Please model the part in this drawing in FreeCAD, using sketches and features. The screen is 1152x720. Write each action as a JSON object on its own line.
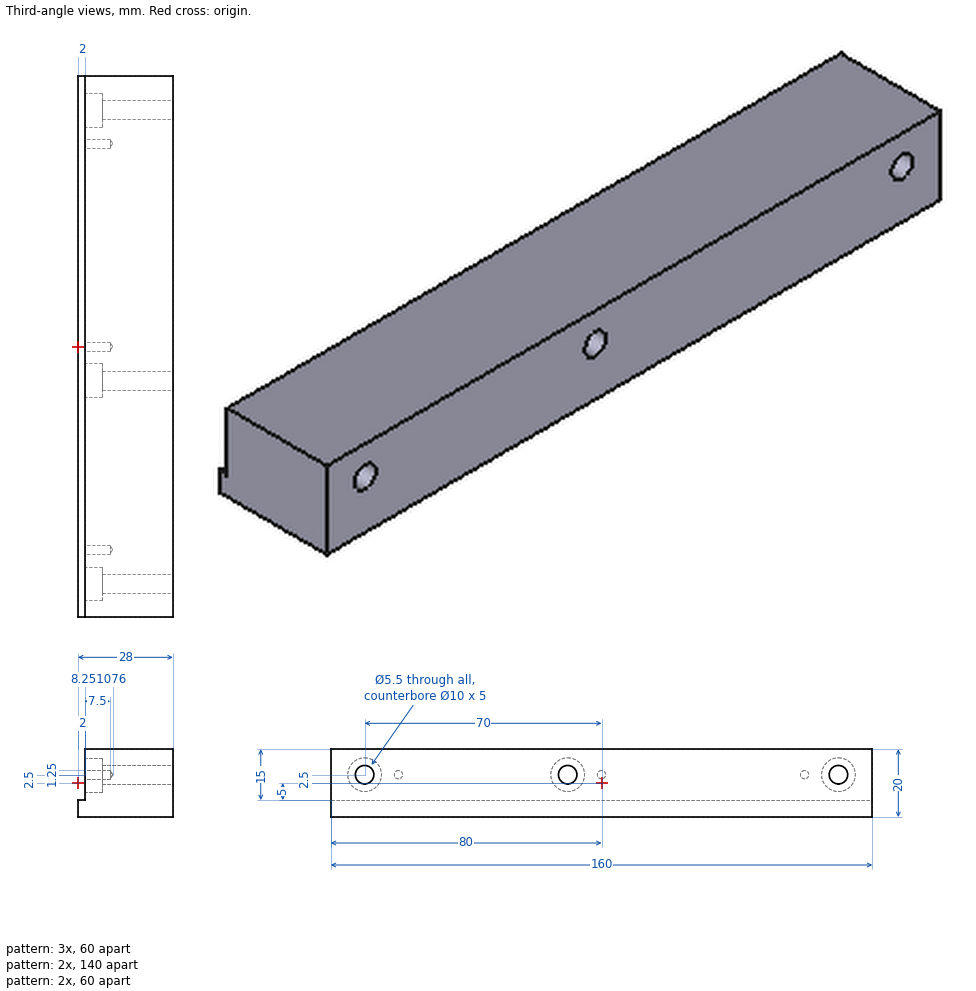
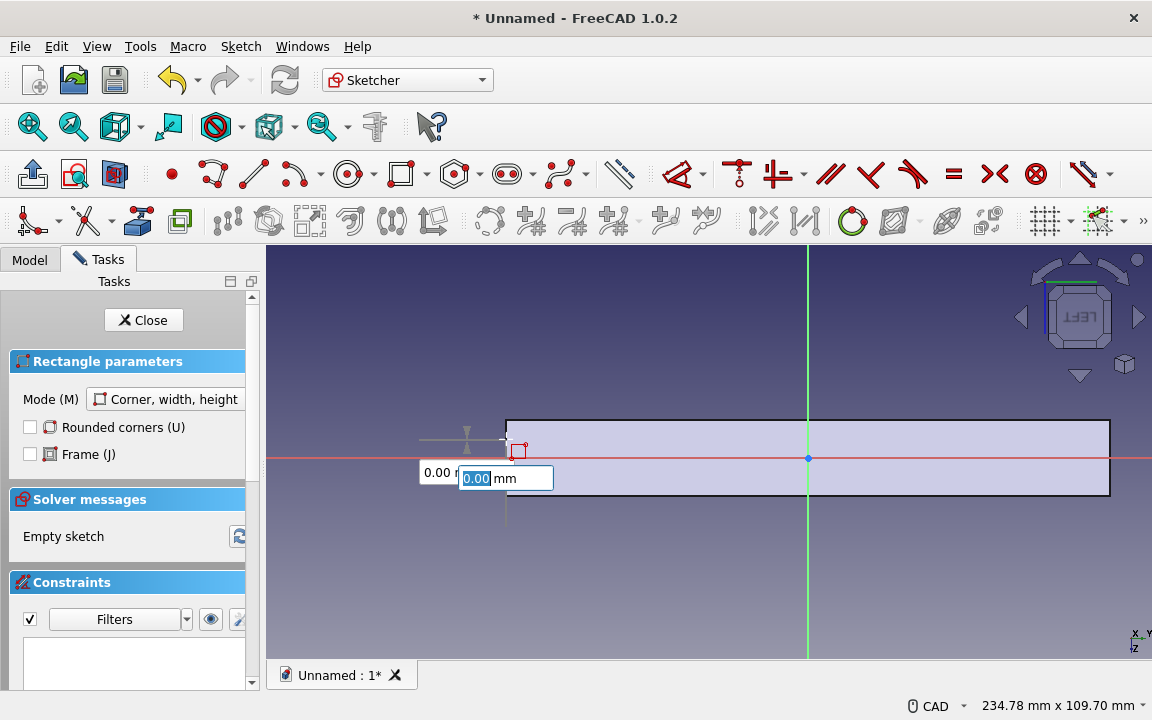
{"action": "scroll", "coordinate": [299, 420], "scroll_direction": "down", "scroll_amount": 2}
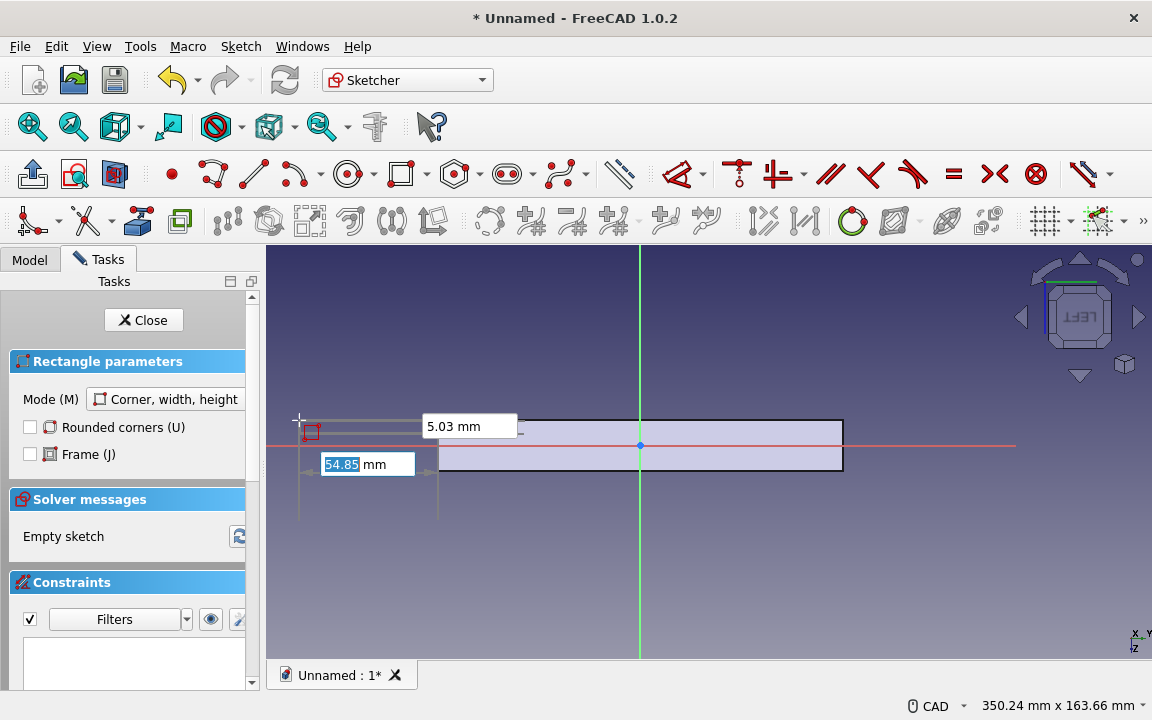
{"action": "left_click", "coordinate": [843, 471]}
{"action": "key", "text": "Escape"}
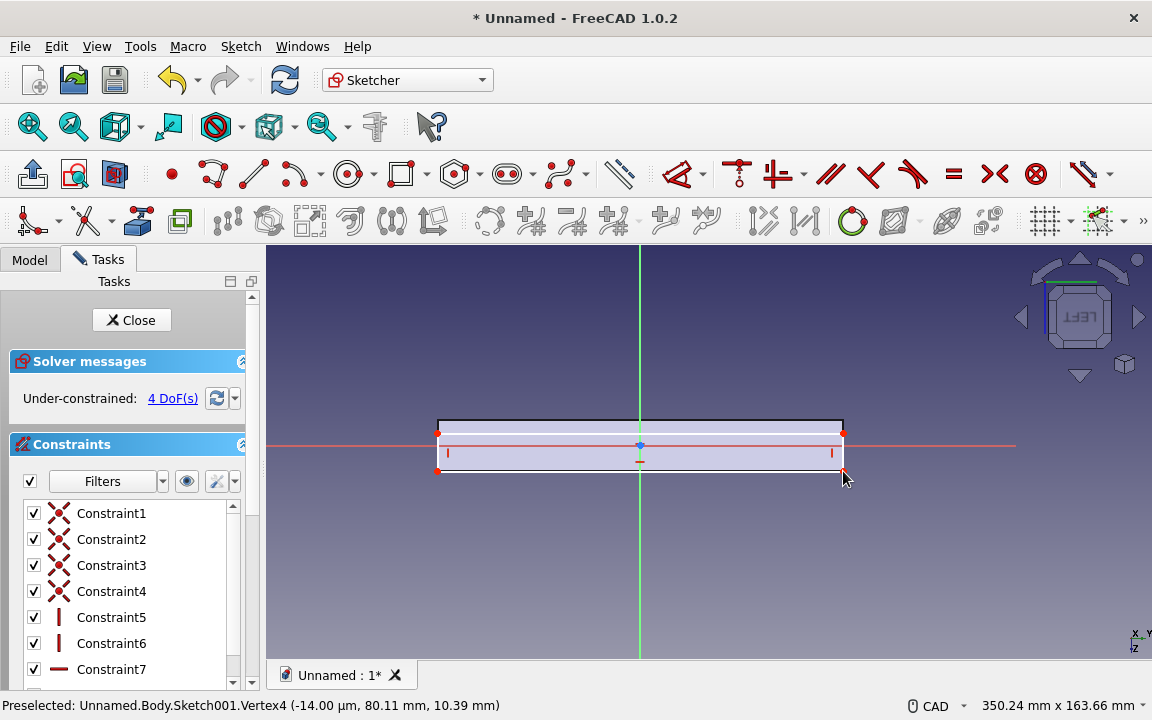
{"action": "key", "text": "d"}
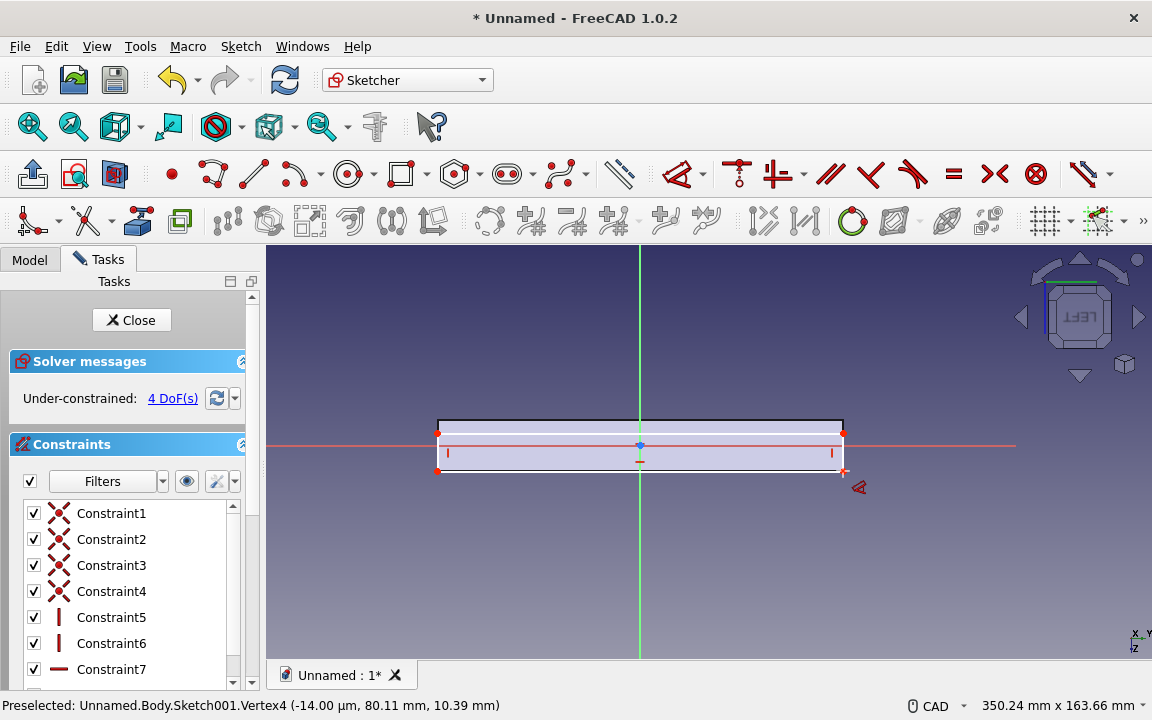
{"action": "left_click", "coordinate": [438, 445]}
{"action": "left_click", "coordinate": [404, 462]}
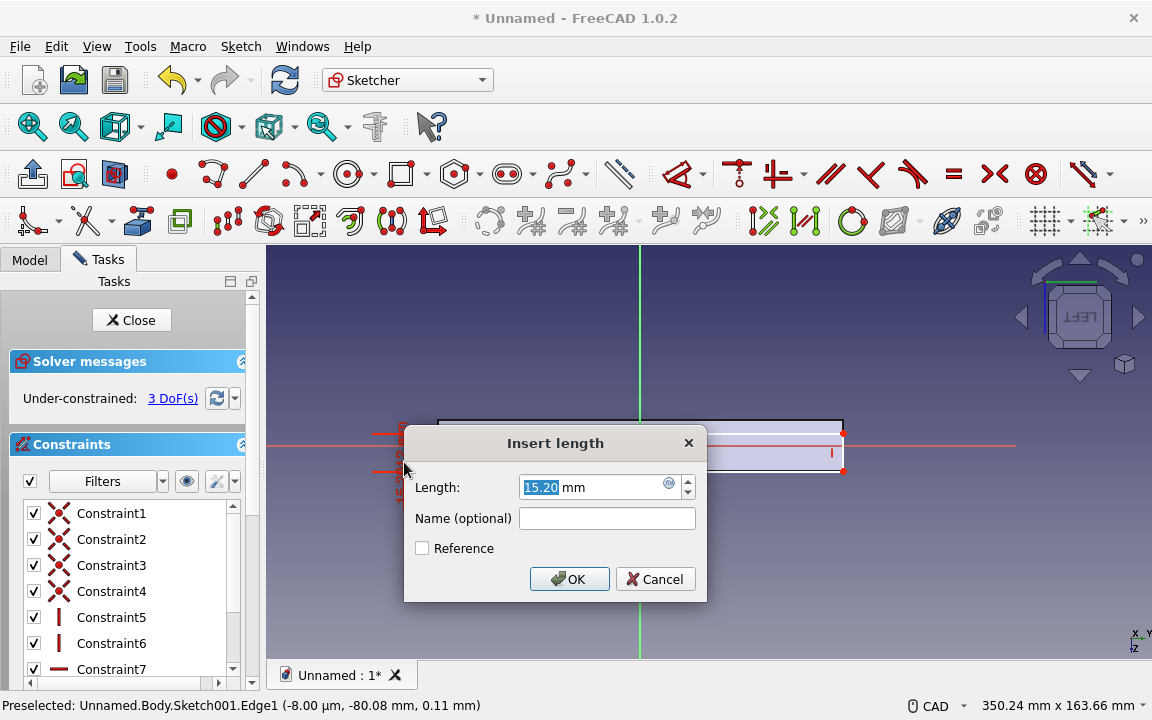
{"action": "type", "text": "15"}
{"action": "key", "text": "Return"}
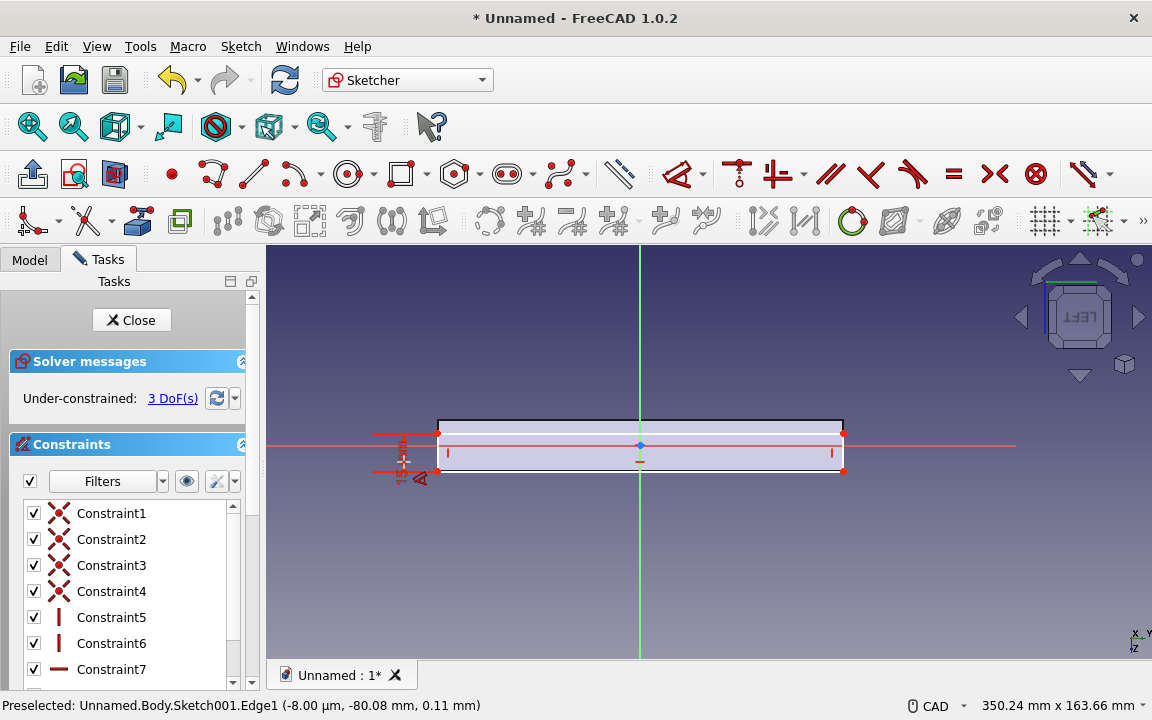
{"action": "scroll", "coordinate": [438, 434], "scroll_direction": "up", "scroll_amount": 6}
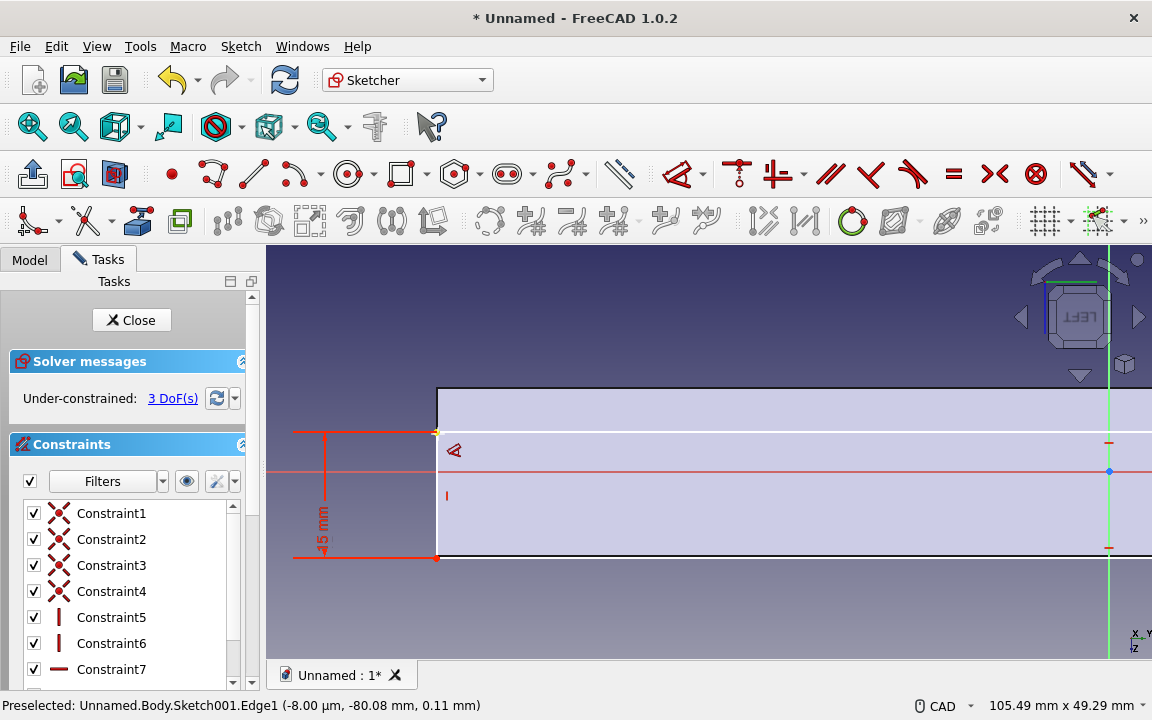
{"action": "left_click", "coordinate": [437, 432]}
{"action": "left_click", "coordinate": [403, 452]}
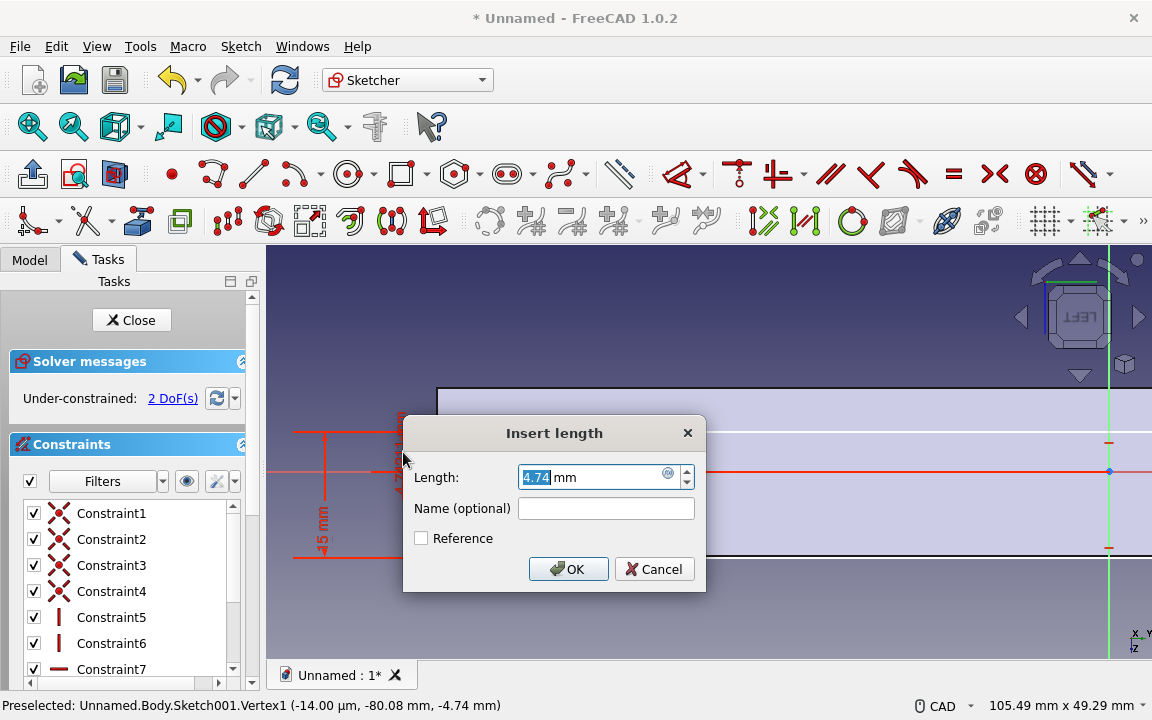
{"action": "type", "text": "5"}
{"action": "key", "text": "Return"}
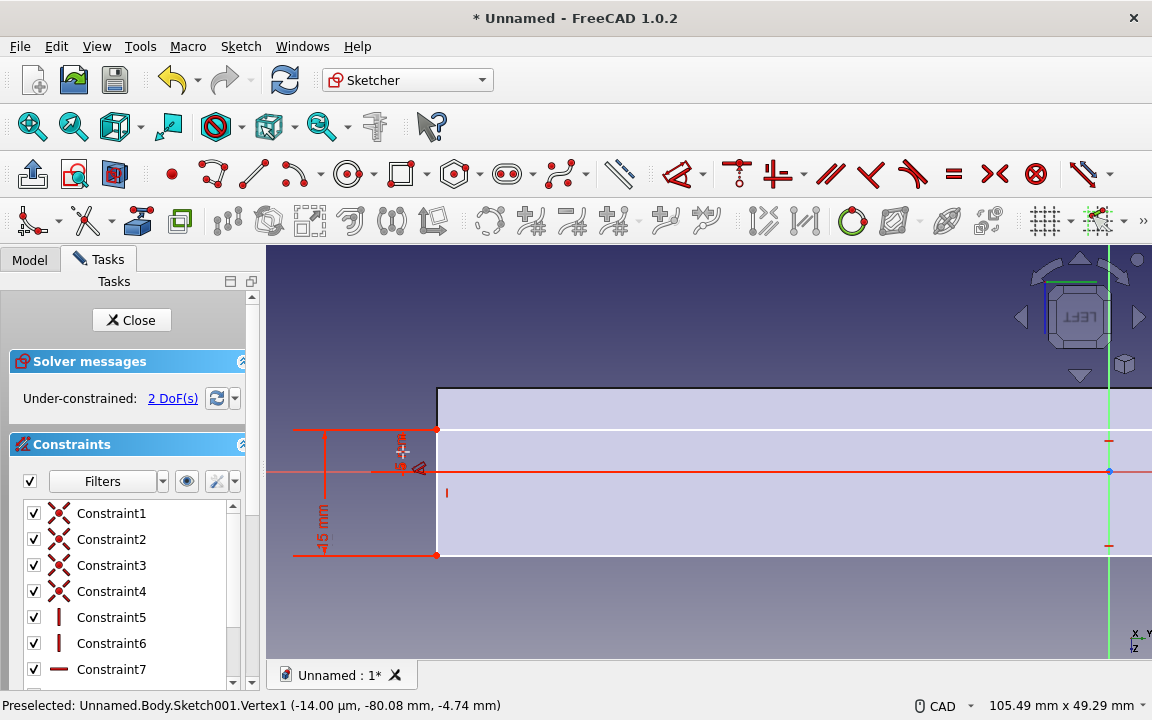
{"action": "left_click", "coordinate": [840, 556]}
{"action": "left_click", "coordinate": [712, 590]}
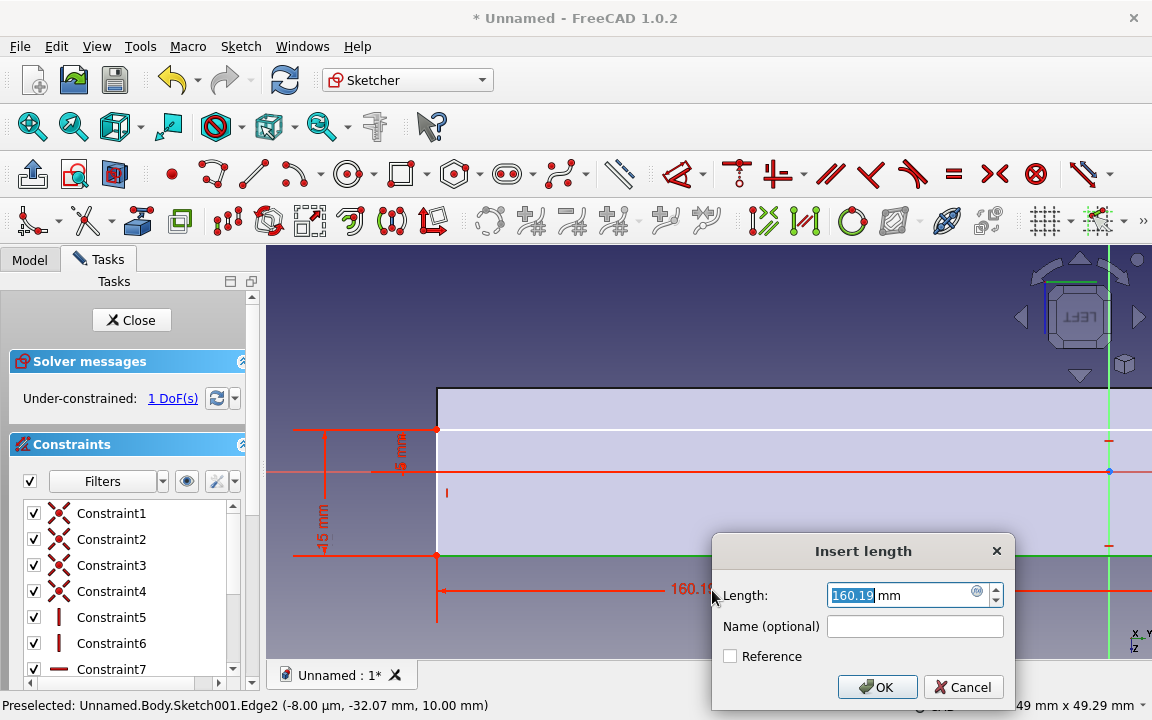
{"action": "type", "text": "160"}
{"action": "key", "text": "Return"}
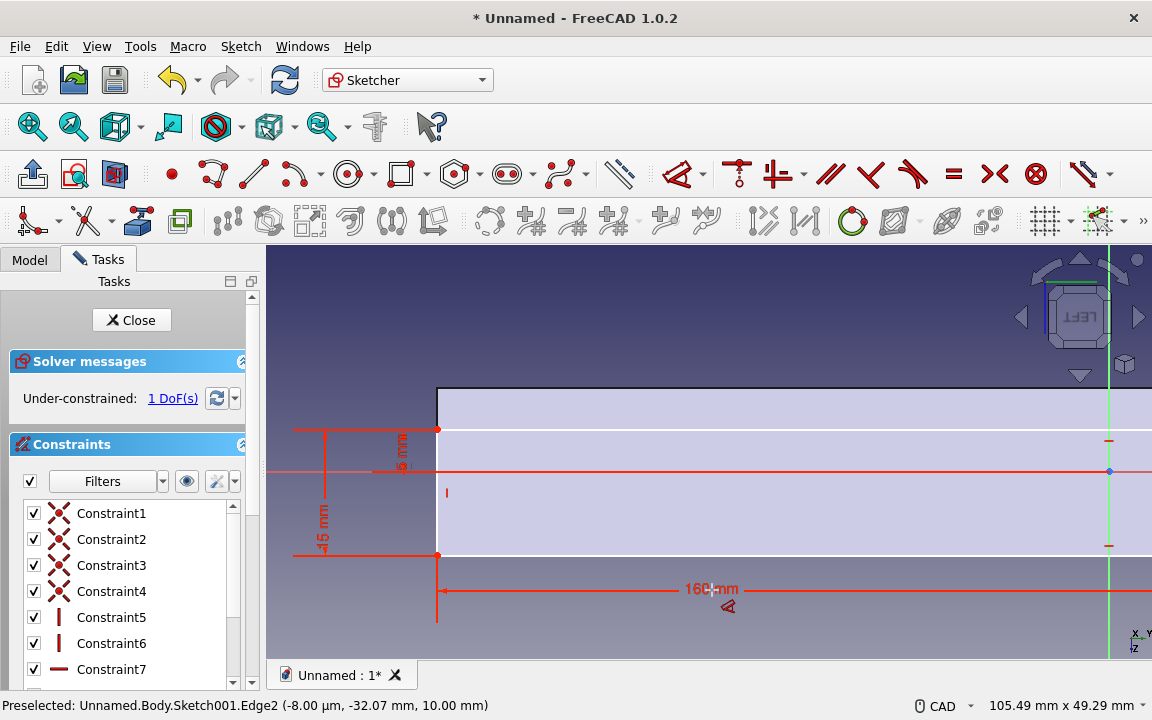
{"action": "left_click", "coordinate": [437, 430]}
{"action": "left_click", "coordinate": [712, 396]}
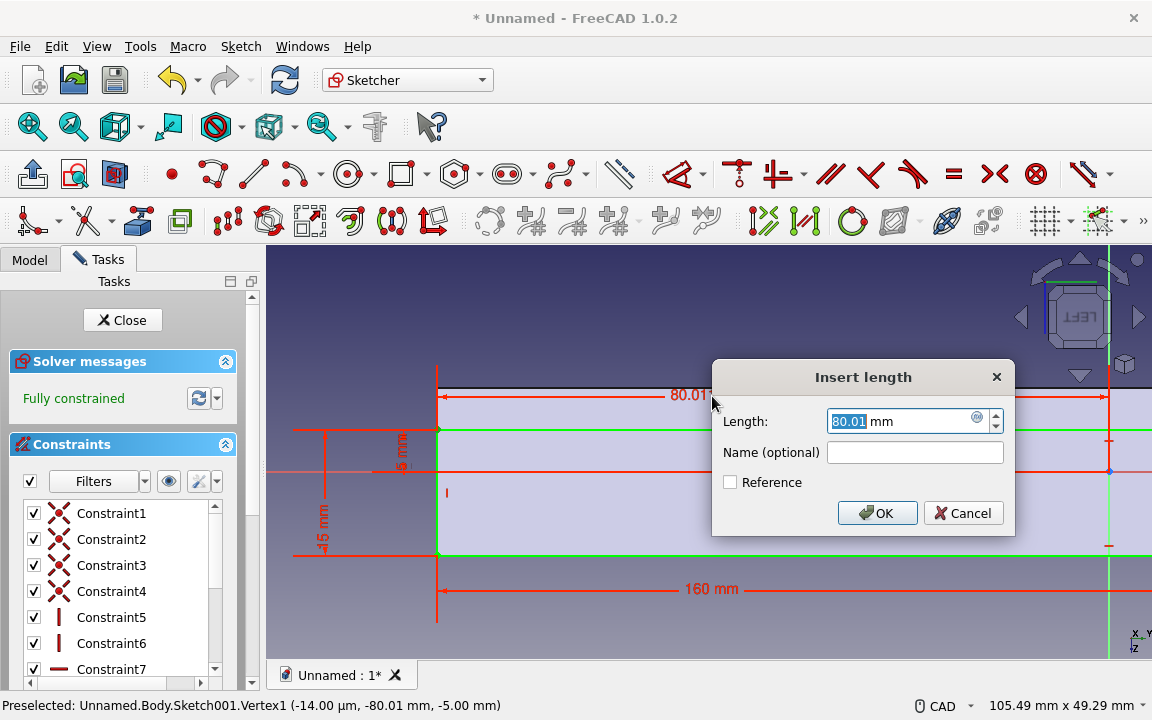
{"action": "type", "text": "80"}
{"action": "key", "text": "Return"}
{"action": "key", "text": "Escape"}